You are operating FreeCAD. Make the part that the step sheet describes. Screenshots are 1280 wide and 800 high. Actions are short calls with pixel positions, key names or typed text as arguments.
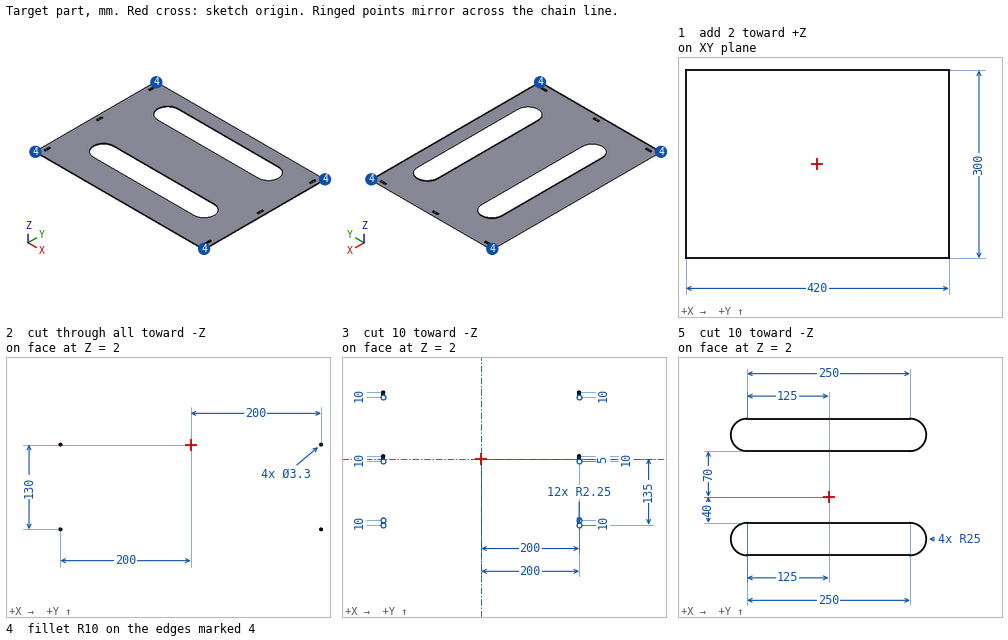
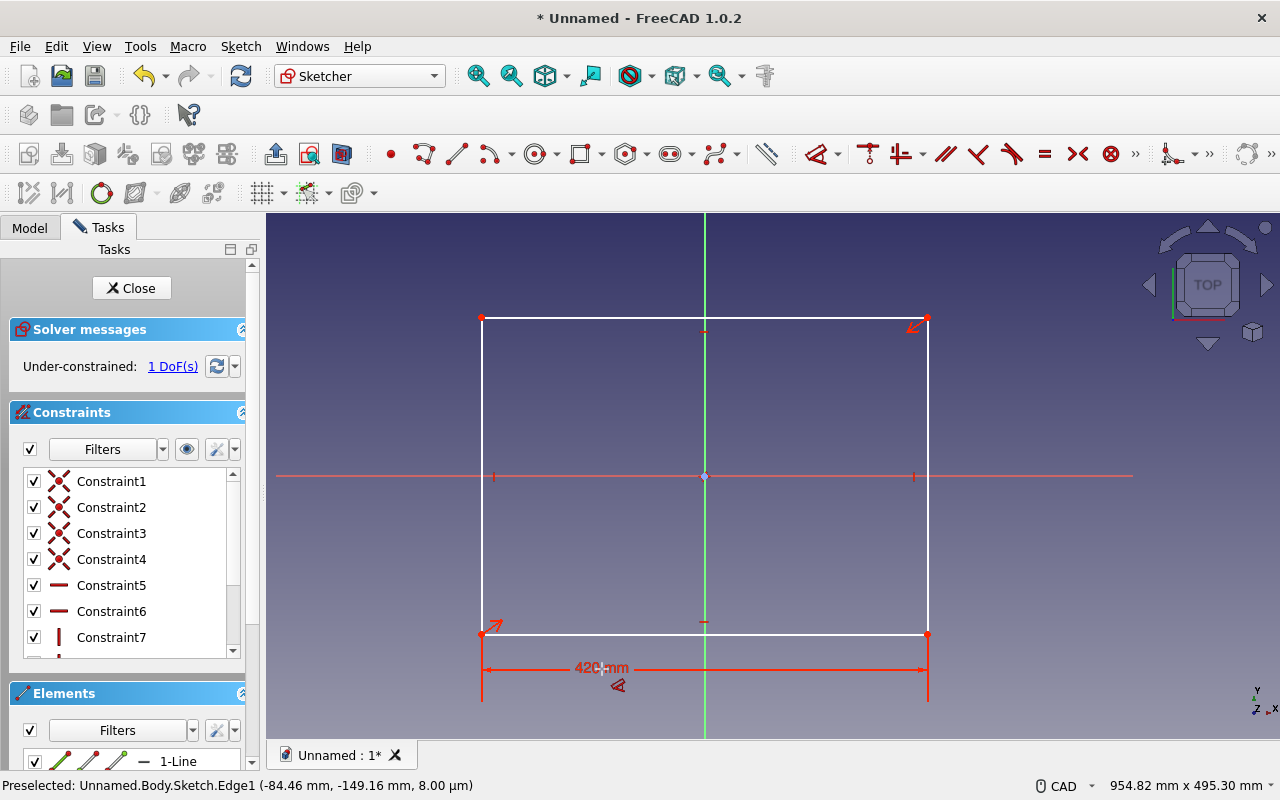
click(928, 540)
click(962, 404)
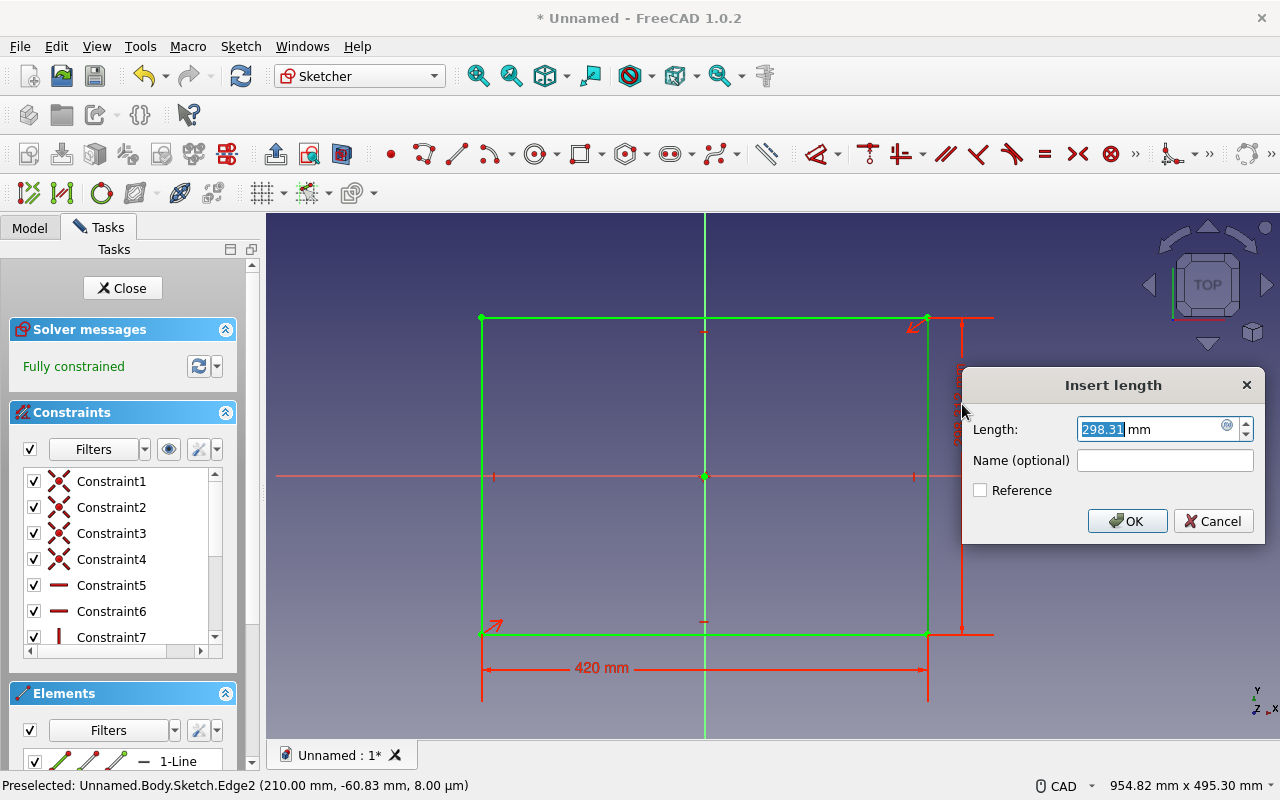
text(300)
key(Return)
key(Escape)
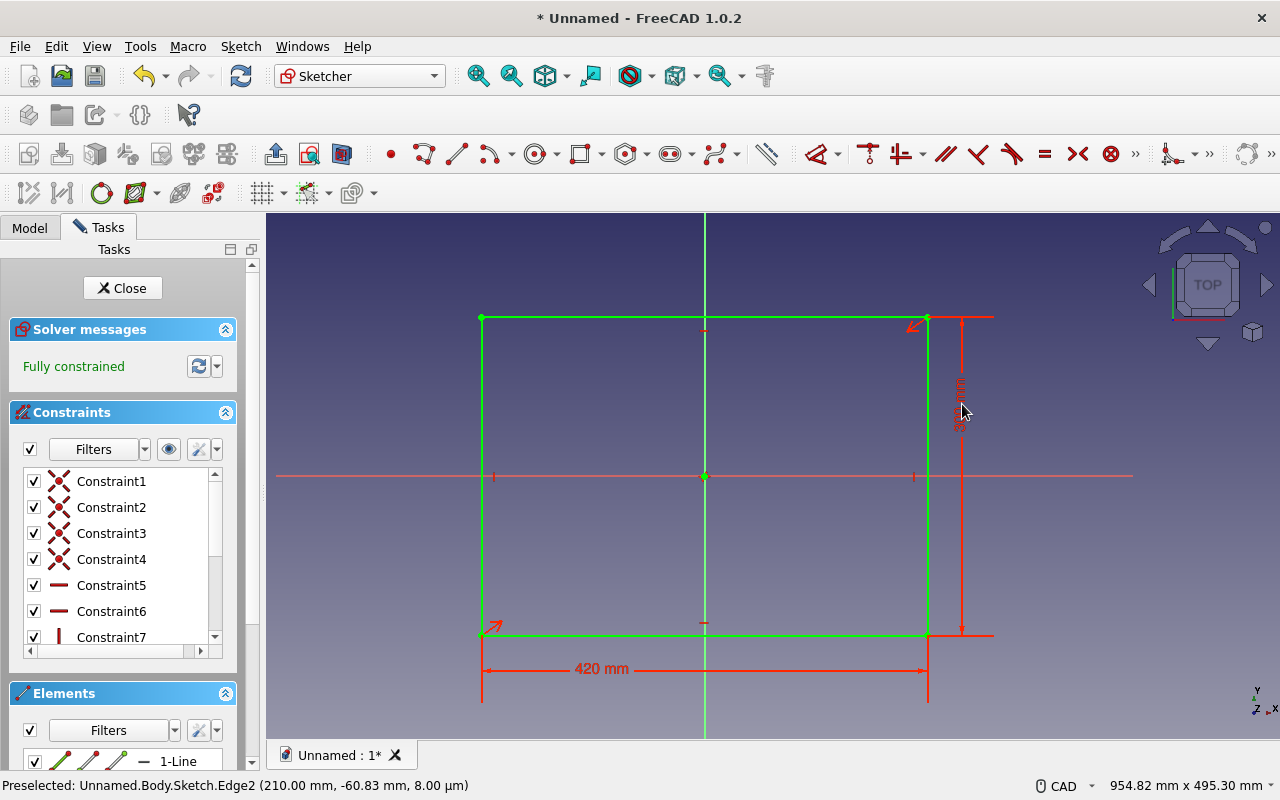
click(123, 288)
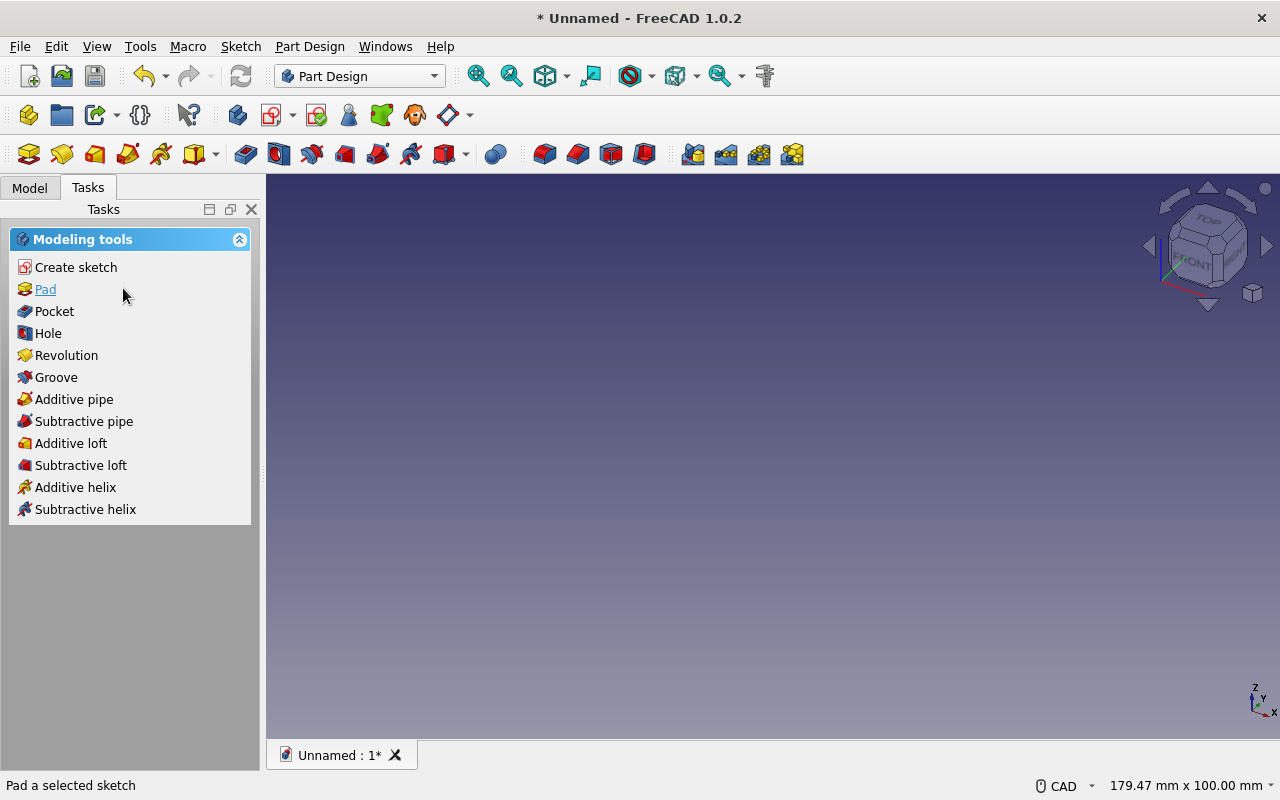
click(29, 154)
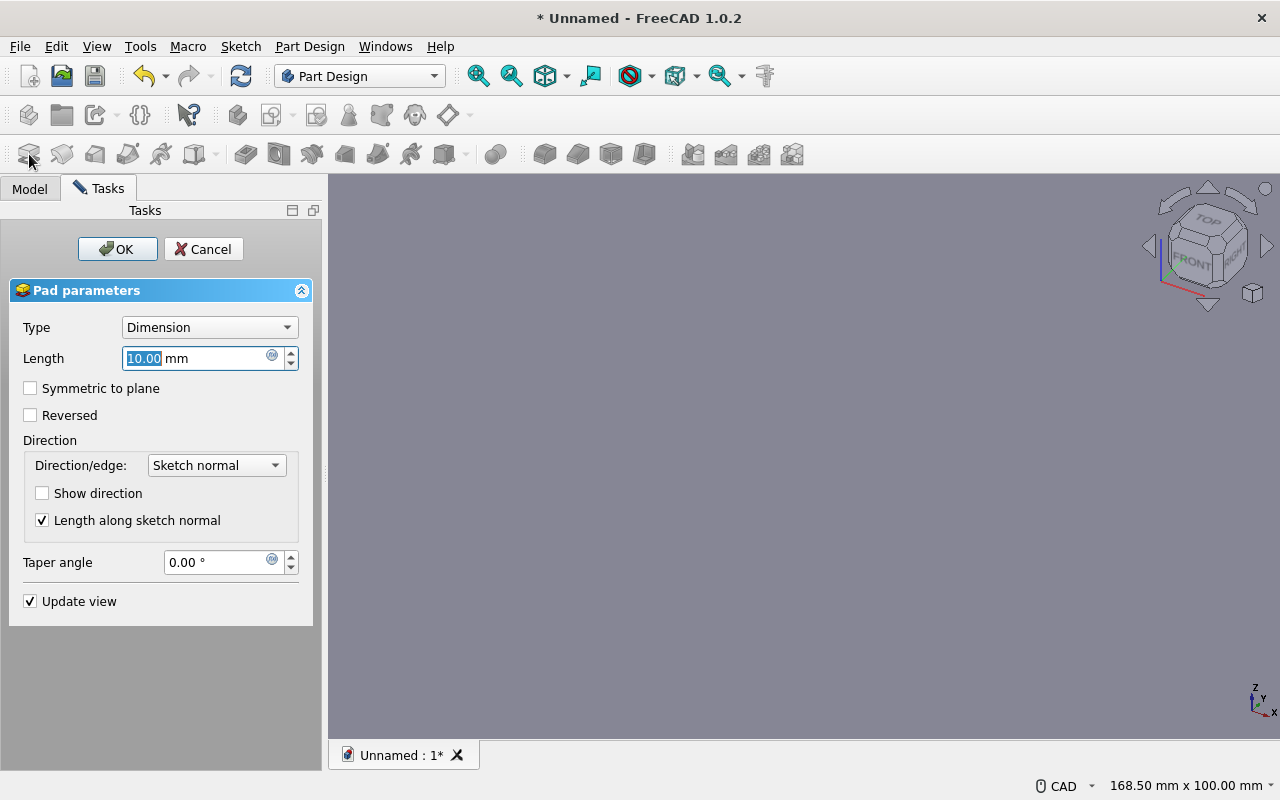
text(2)
key(Tab)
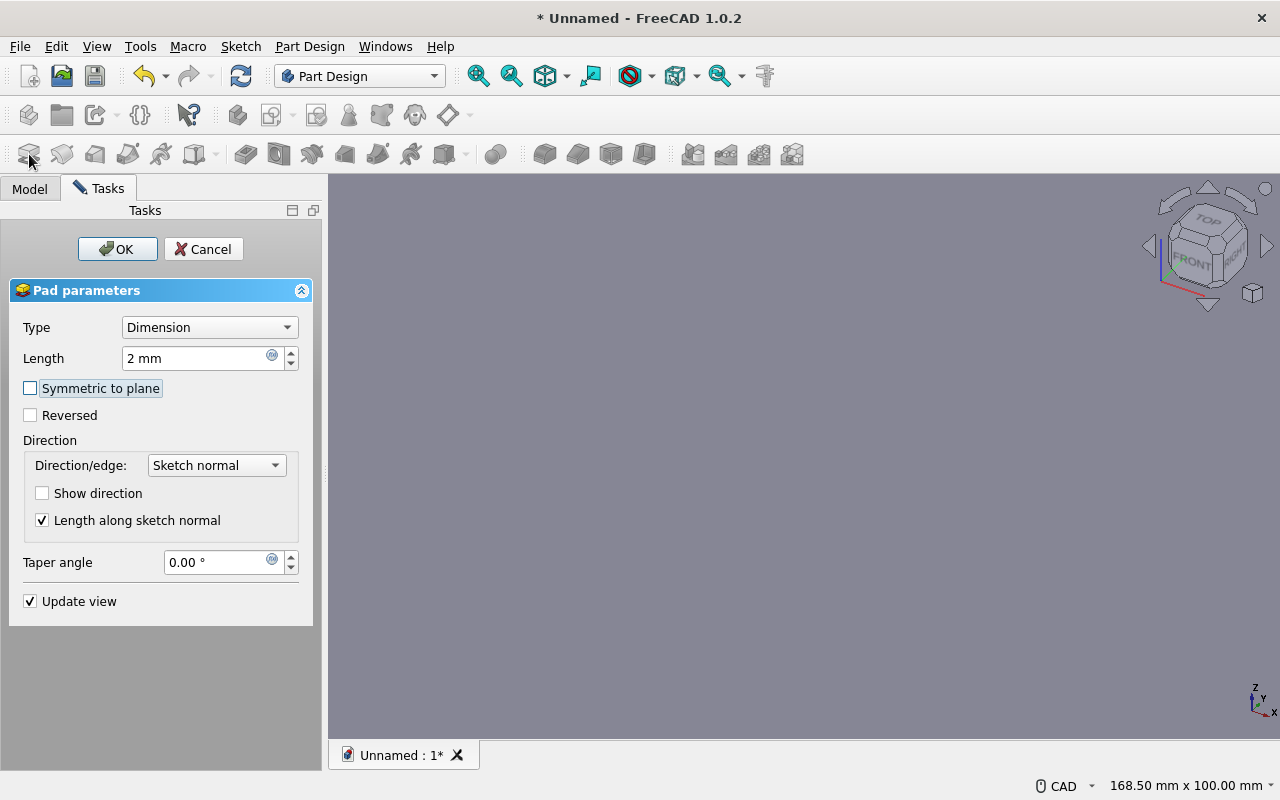
click(118, 249)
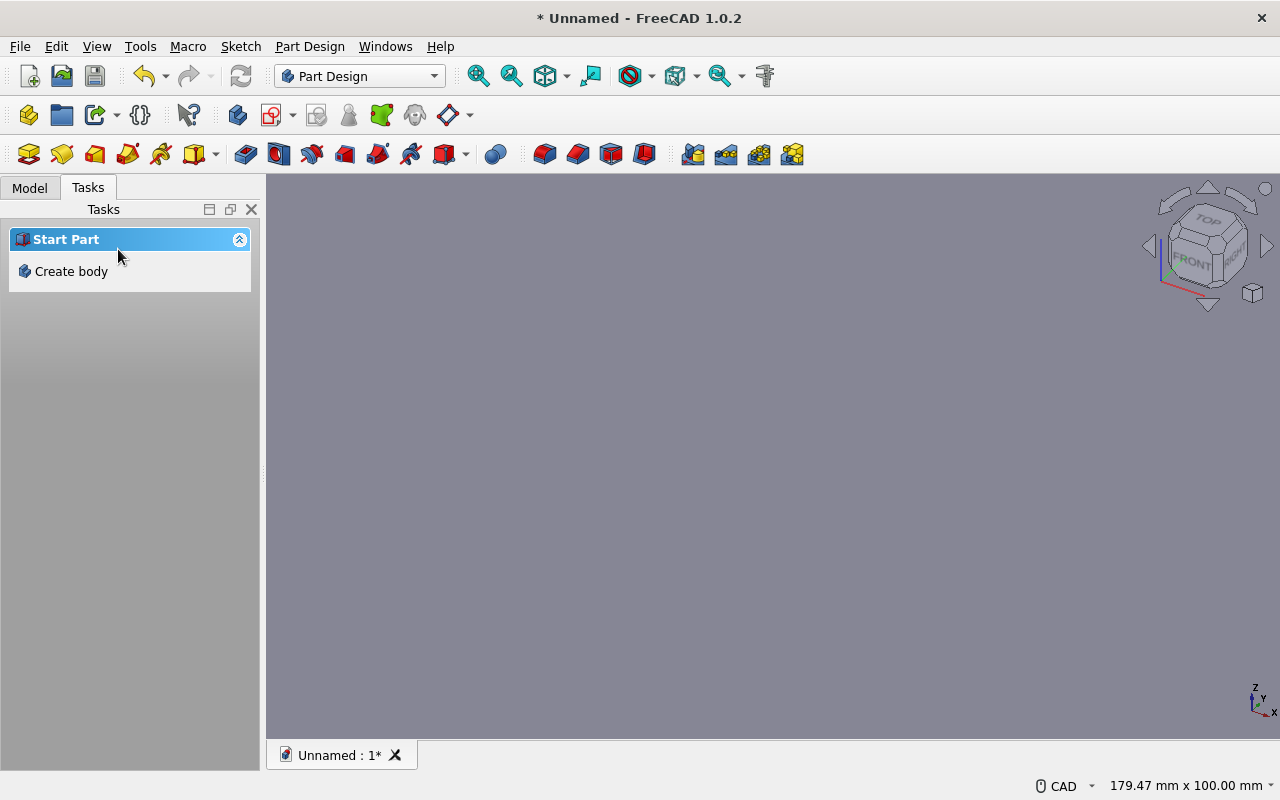
click(479, 76)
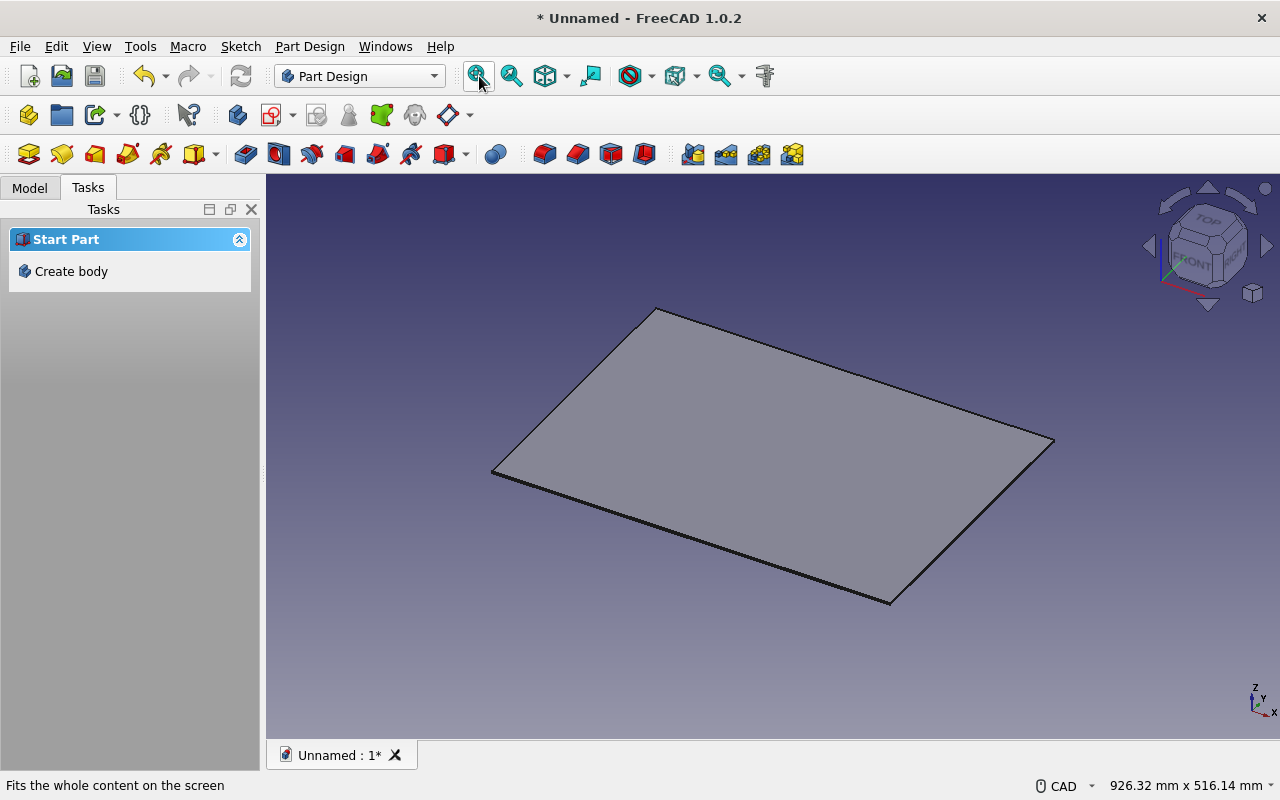
click(830, 473)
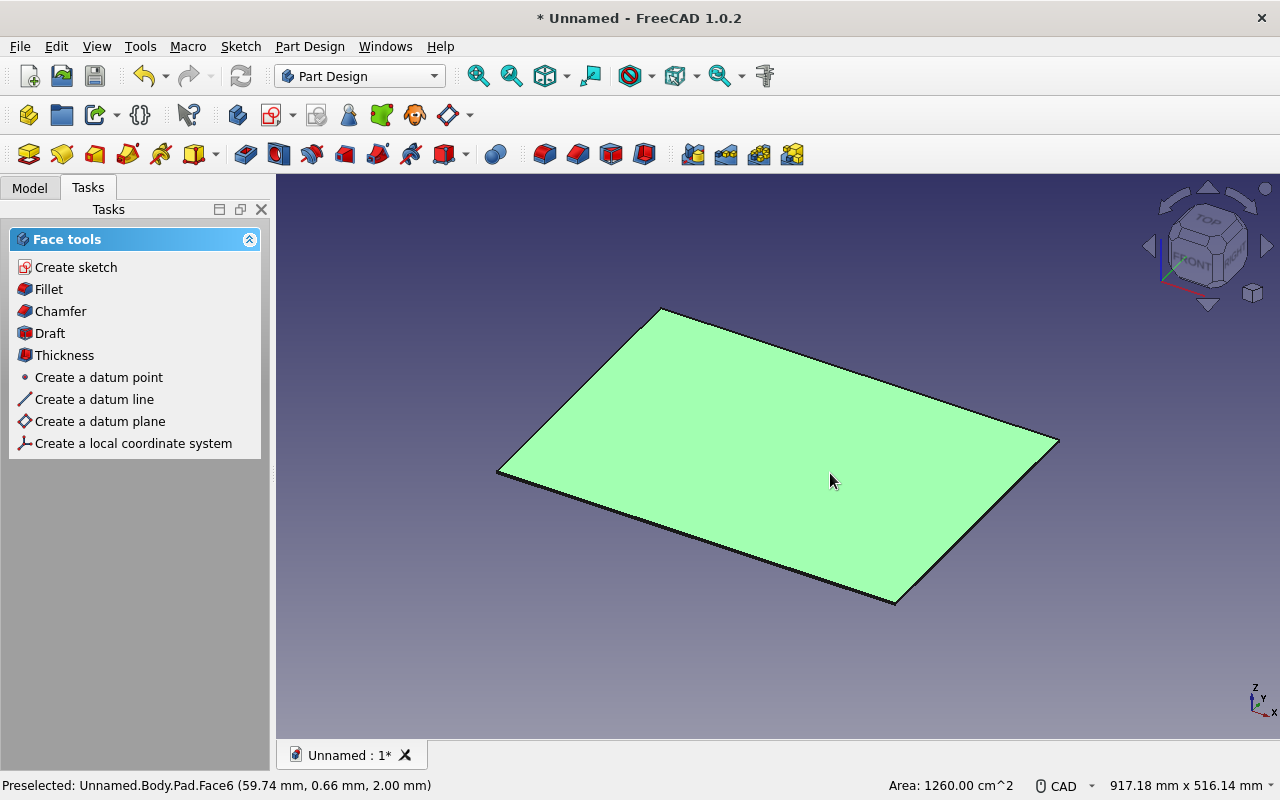
click(270, 116)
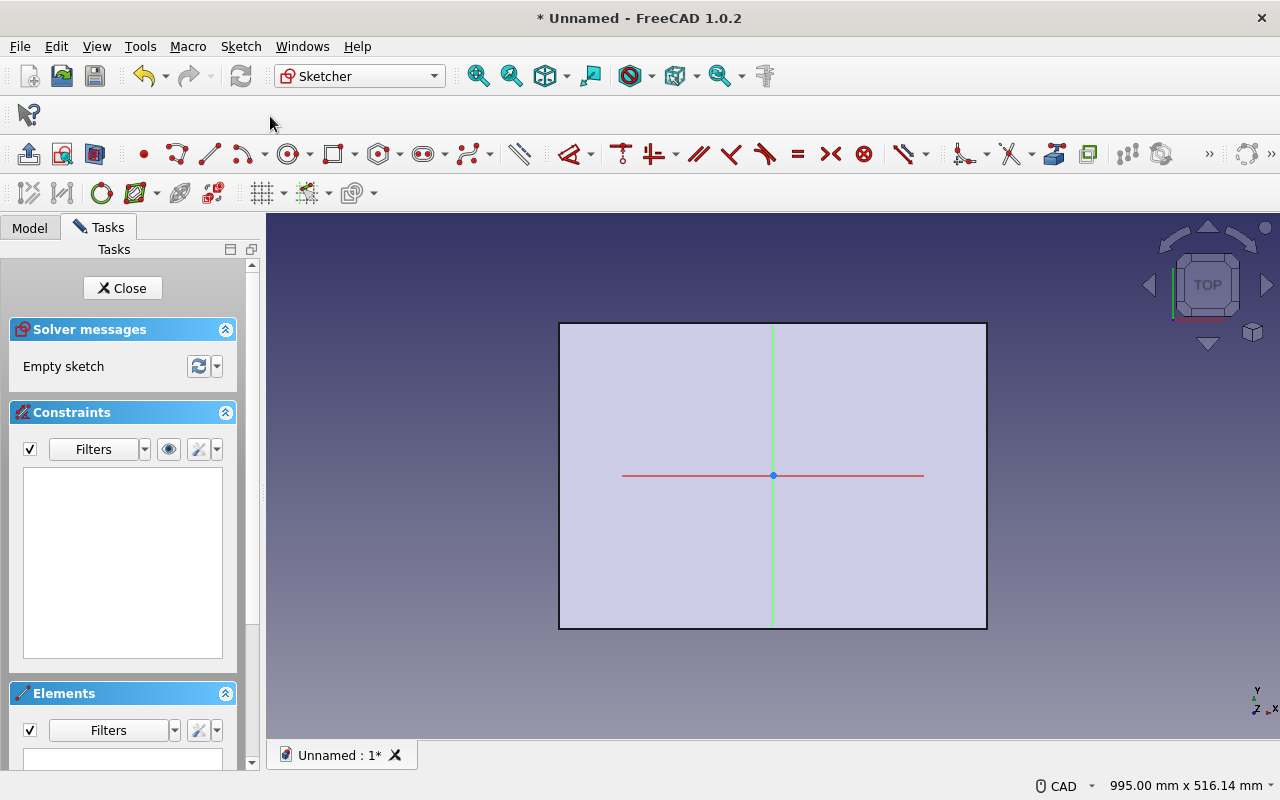
scroll(912, 677, up, 2)